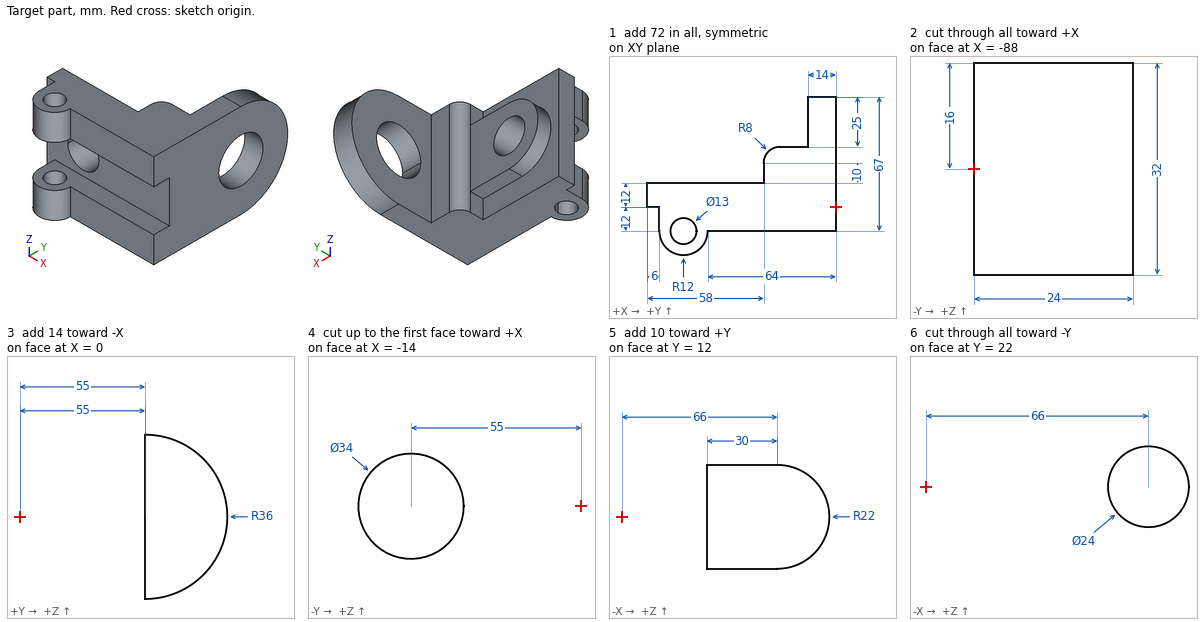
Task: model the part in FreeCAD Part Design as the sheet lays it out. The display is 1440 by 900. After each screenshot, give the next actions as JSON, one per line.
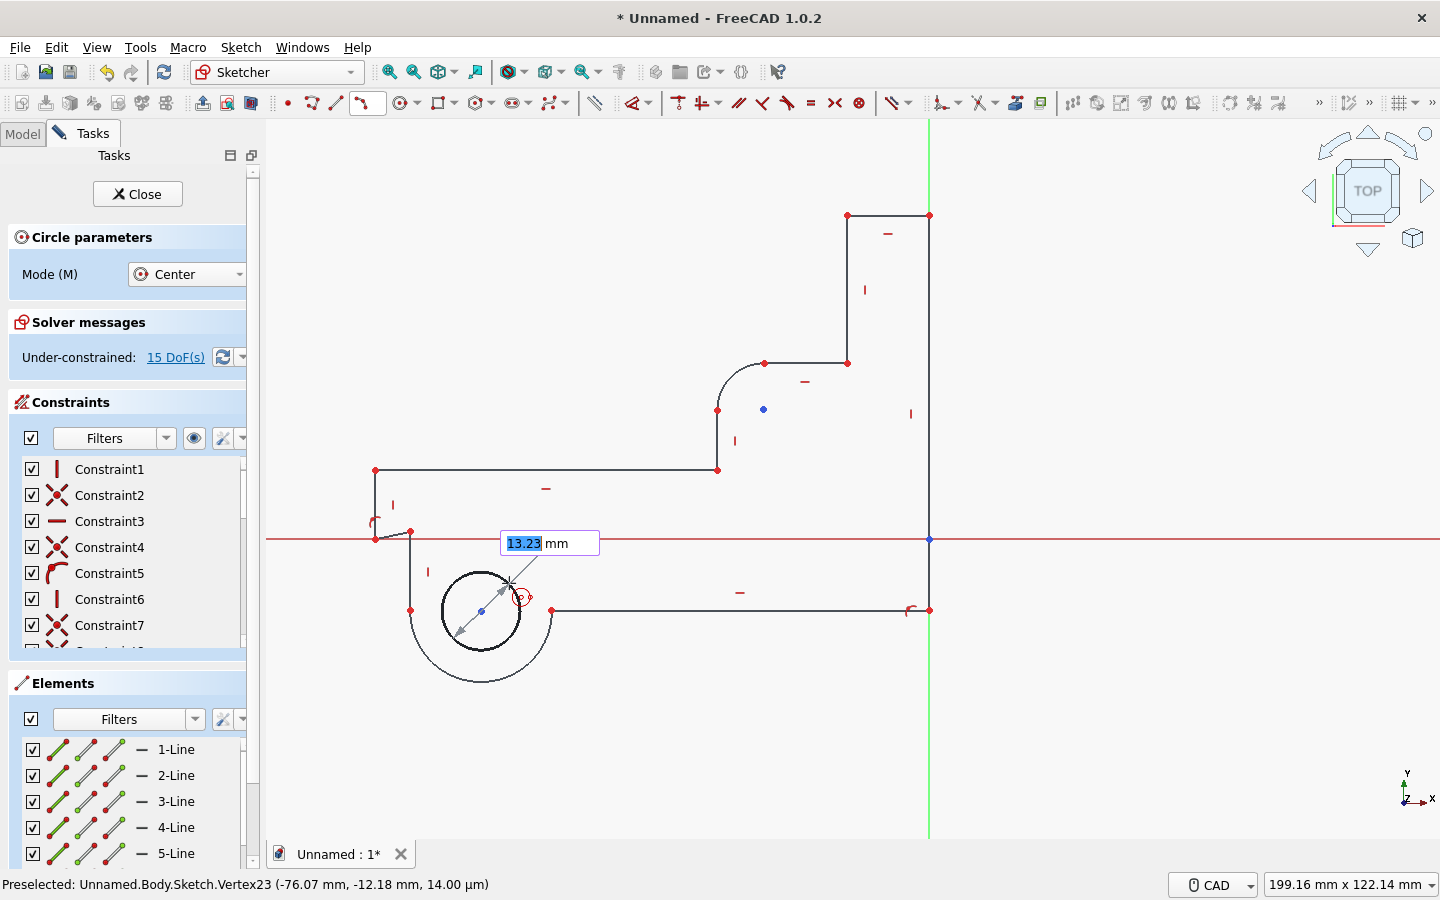
{"action": "type", "text": "13"}
{"action": "key", "text": "Return"}
{"action": "key", "text": "Escape"}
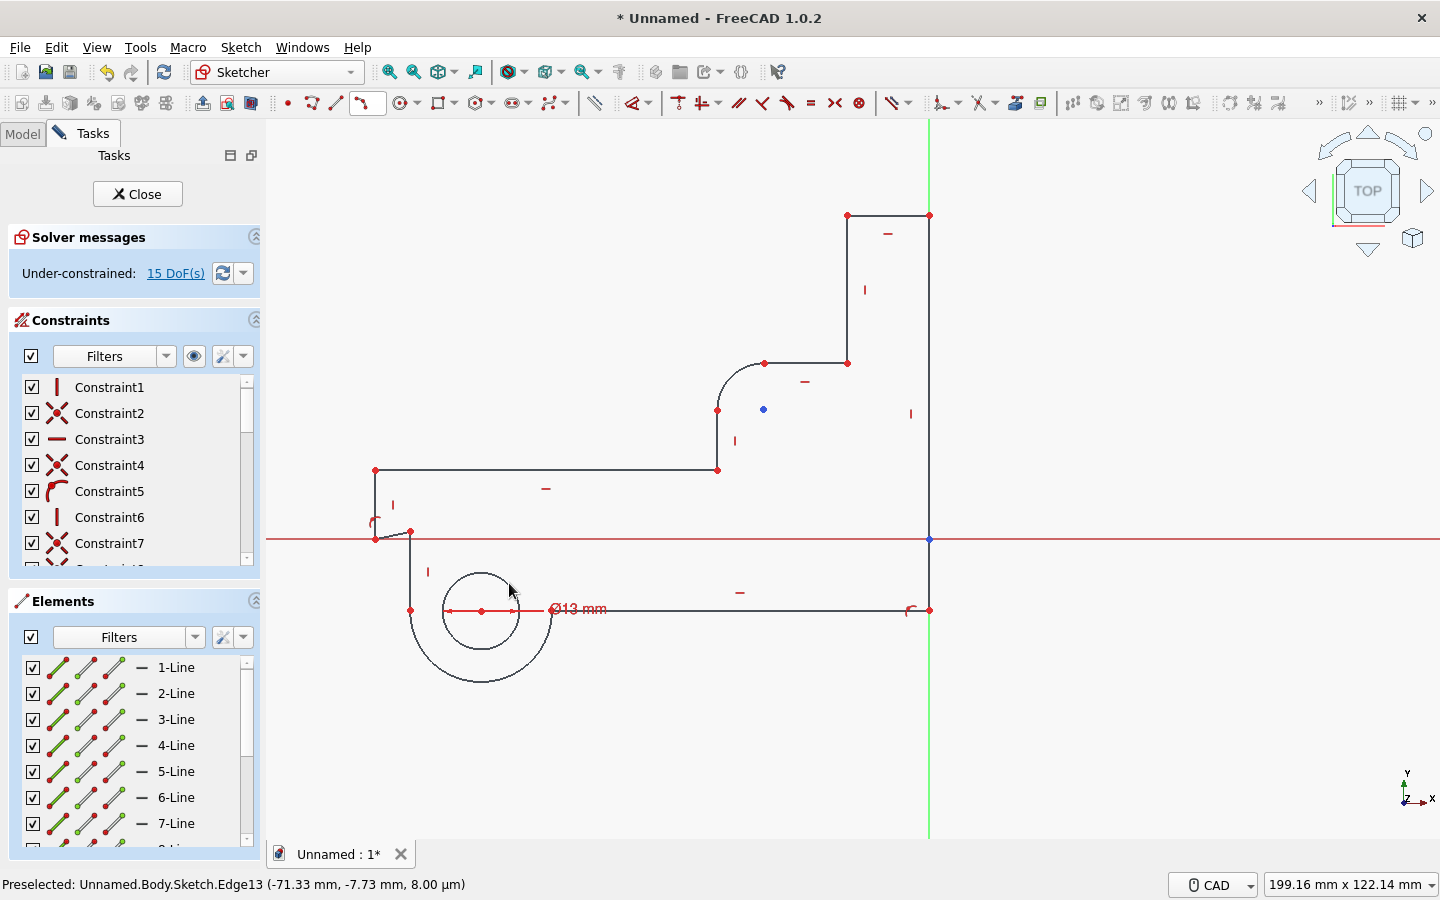
{"action": "left_click", "coordinate": [717, 428]}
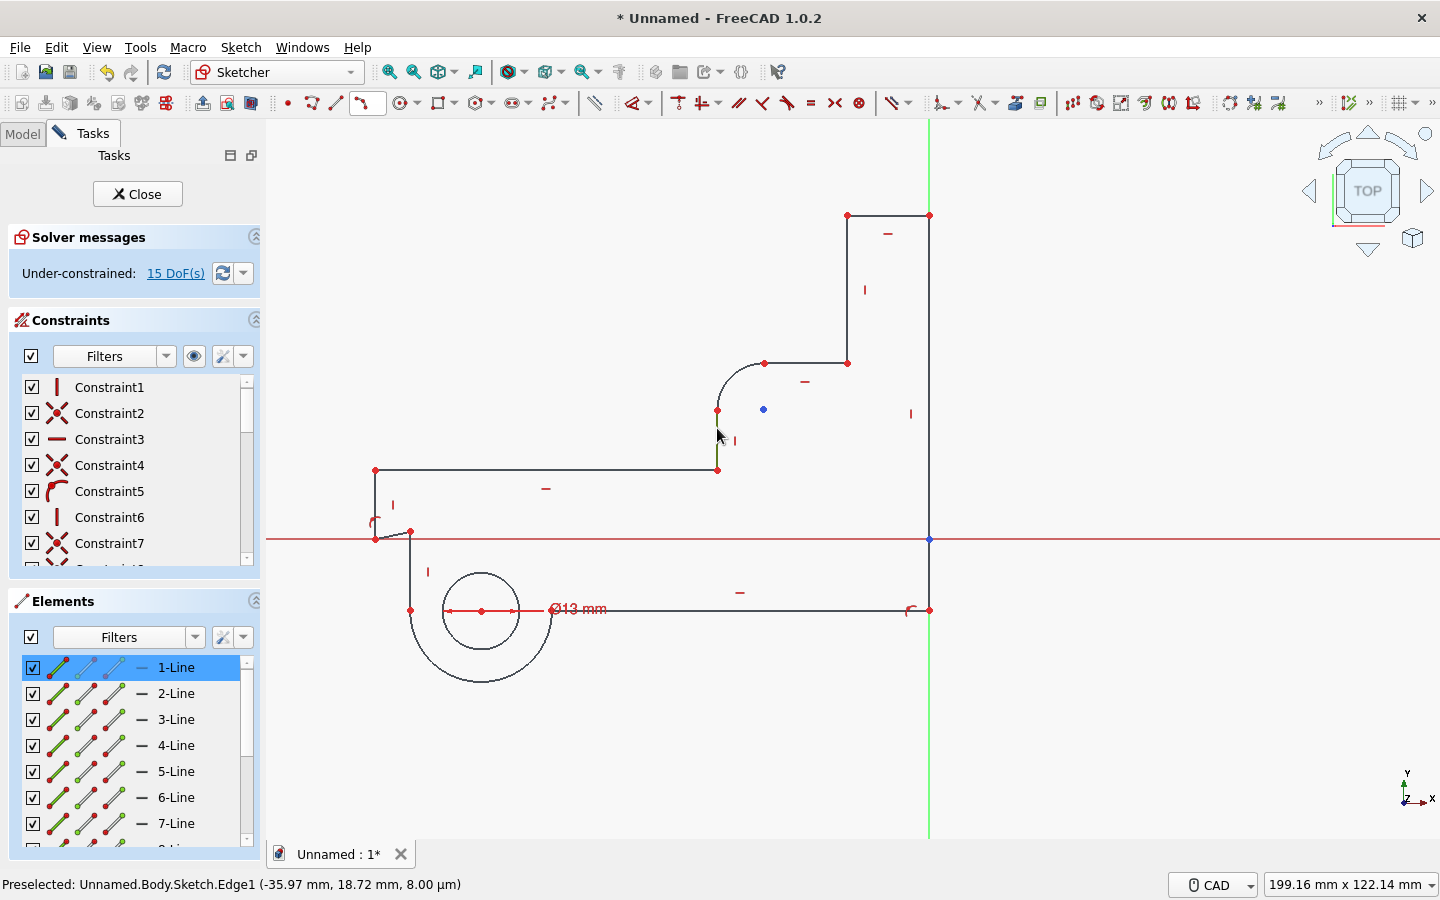
{"action": "left_click", "coordinate": [743, 368]}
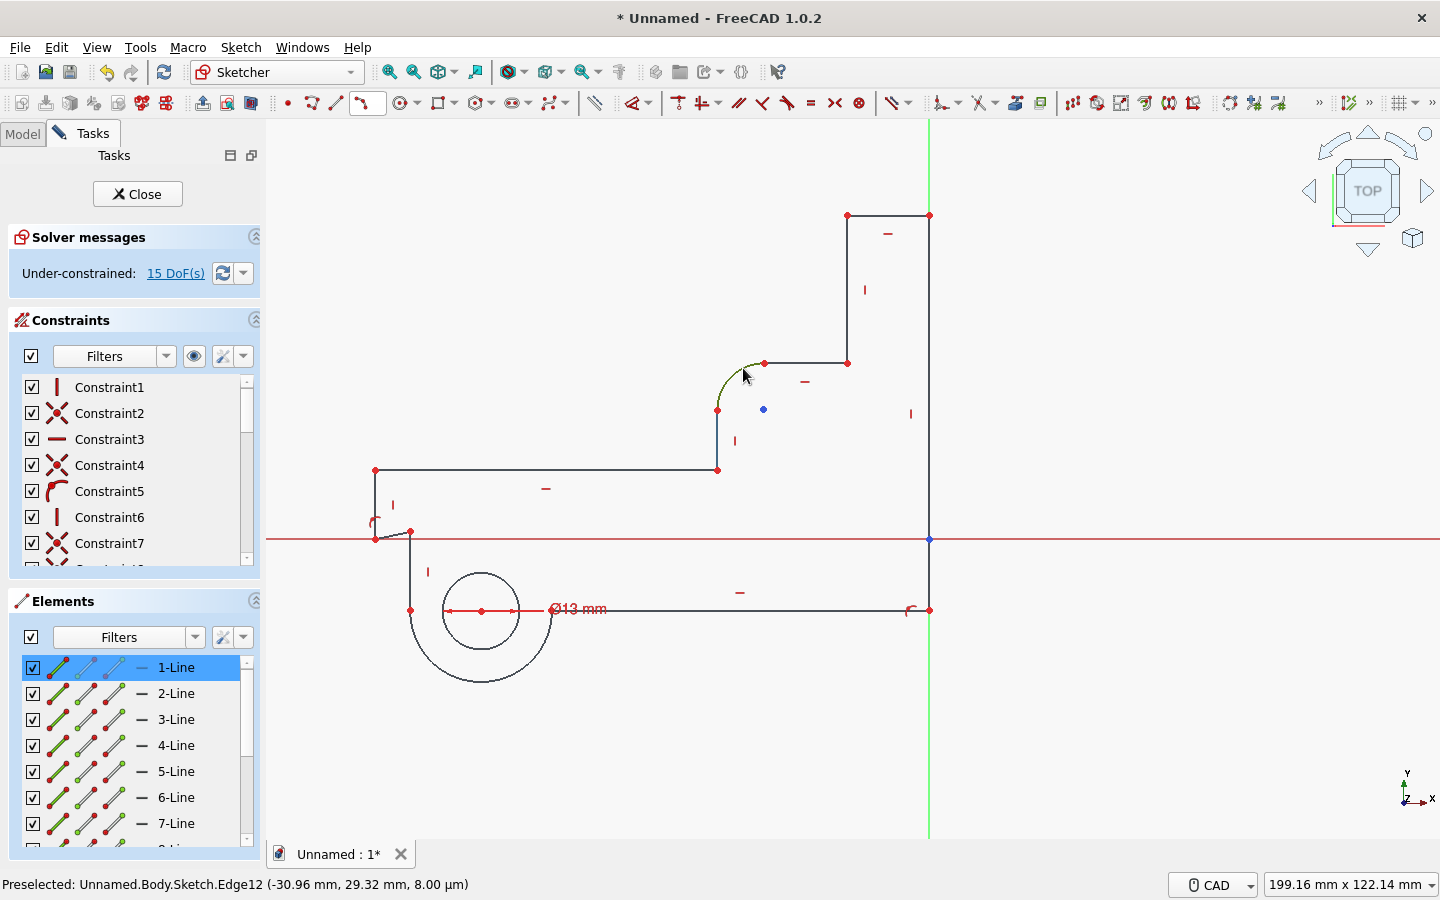
{"action": "left_click", "coordinate": [788, 104]}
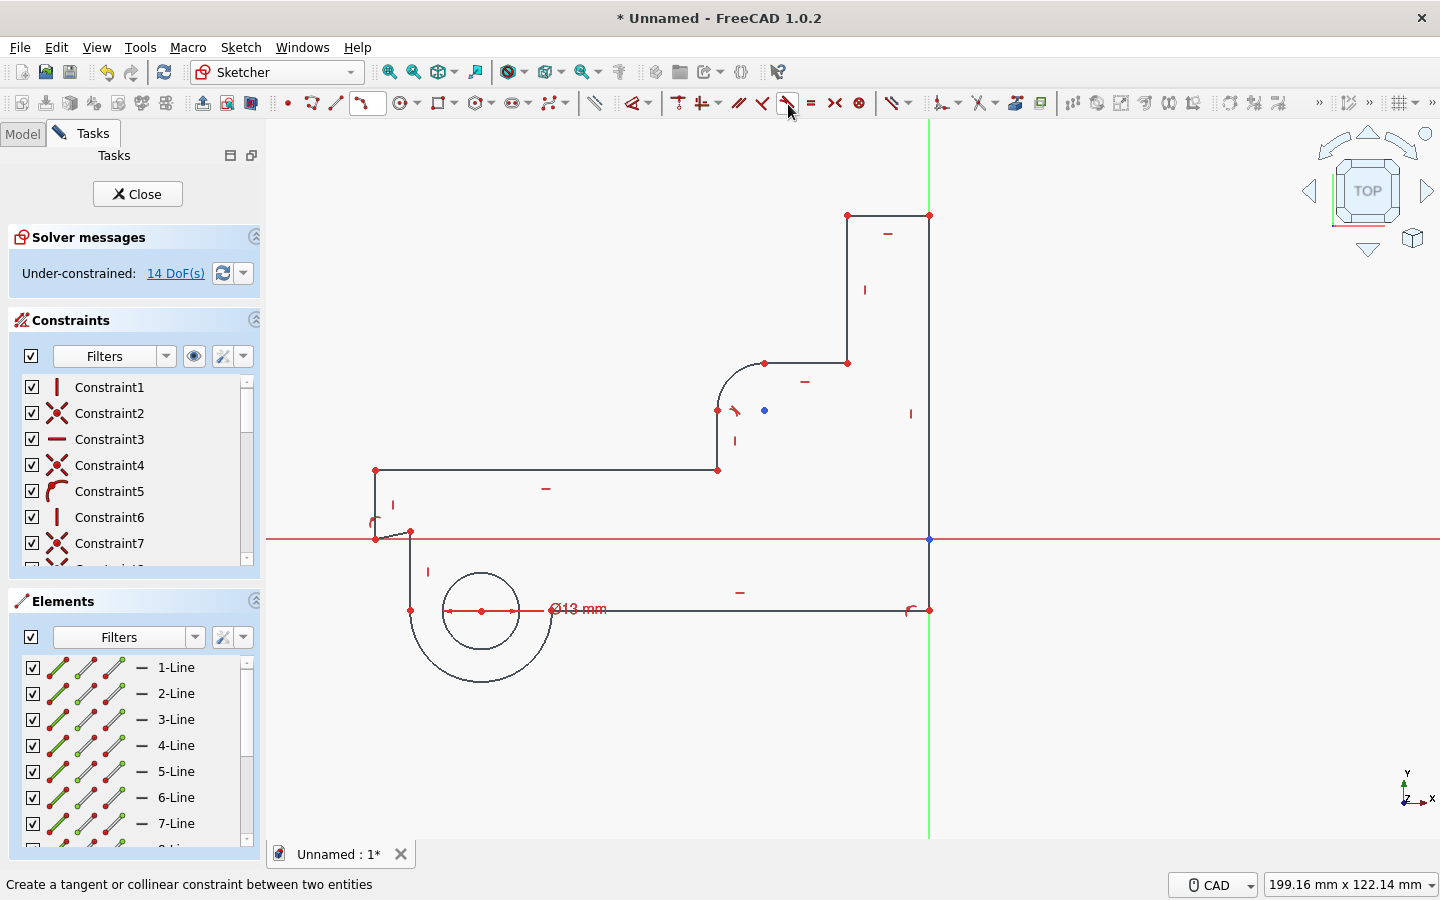
{"action": "left_click", "coordinate": [410, 555]}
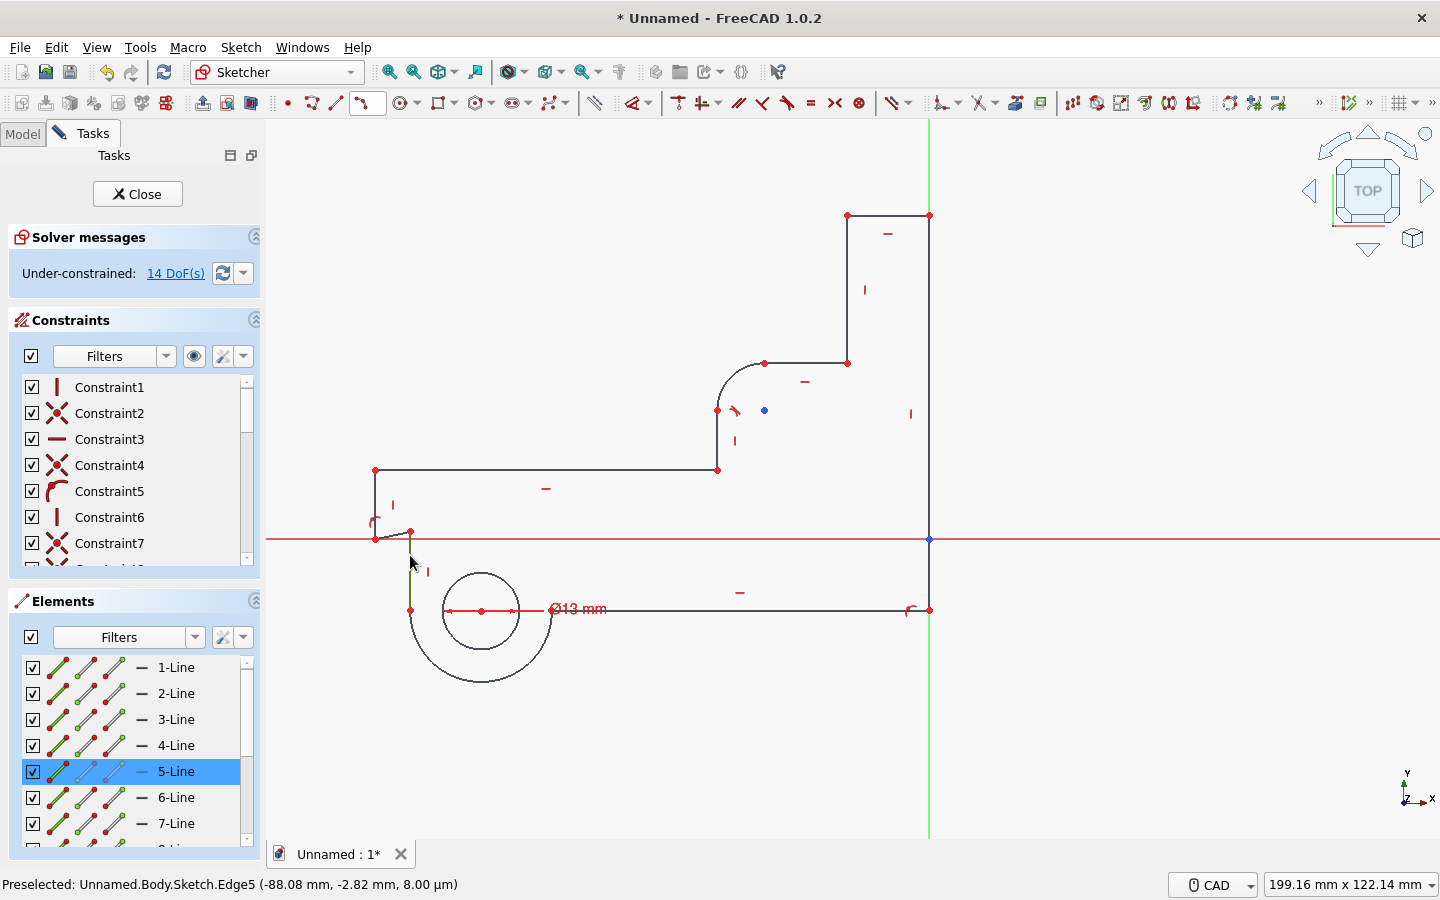
{"action": "left_click", "coordinate": [439, 668]}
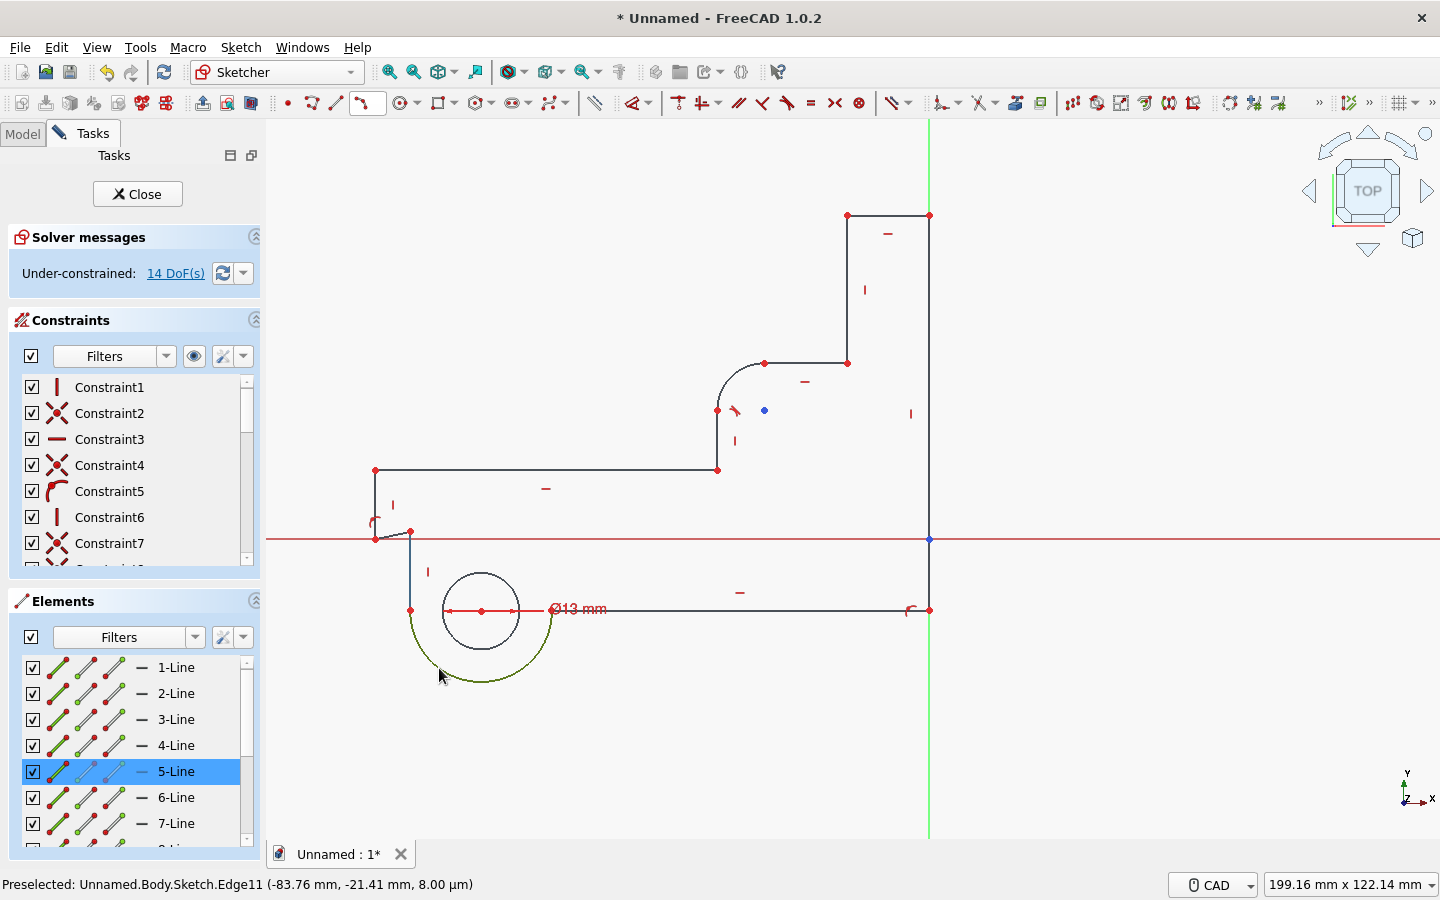
{"action": "left_click", "coordinate": [788, 104]}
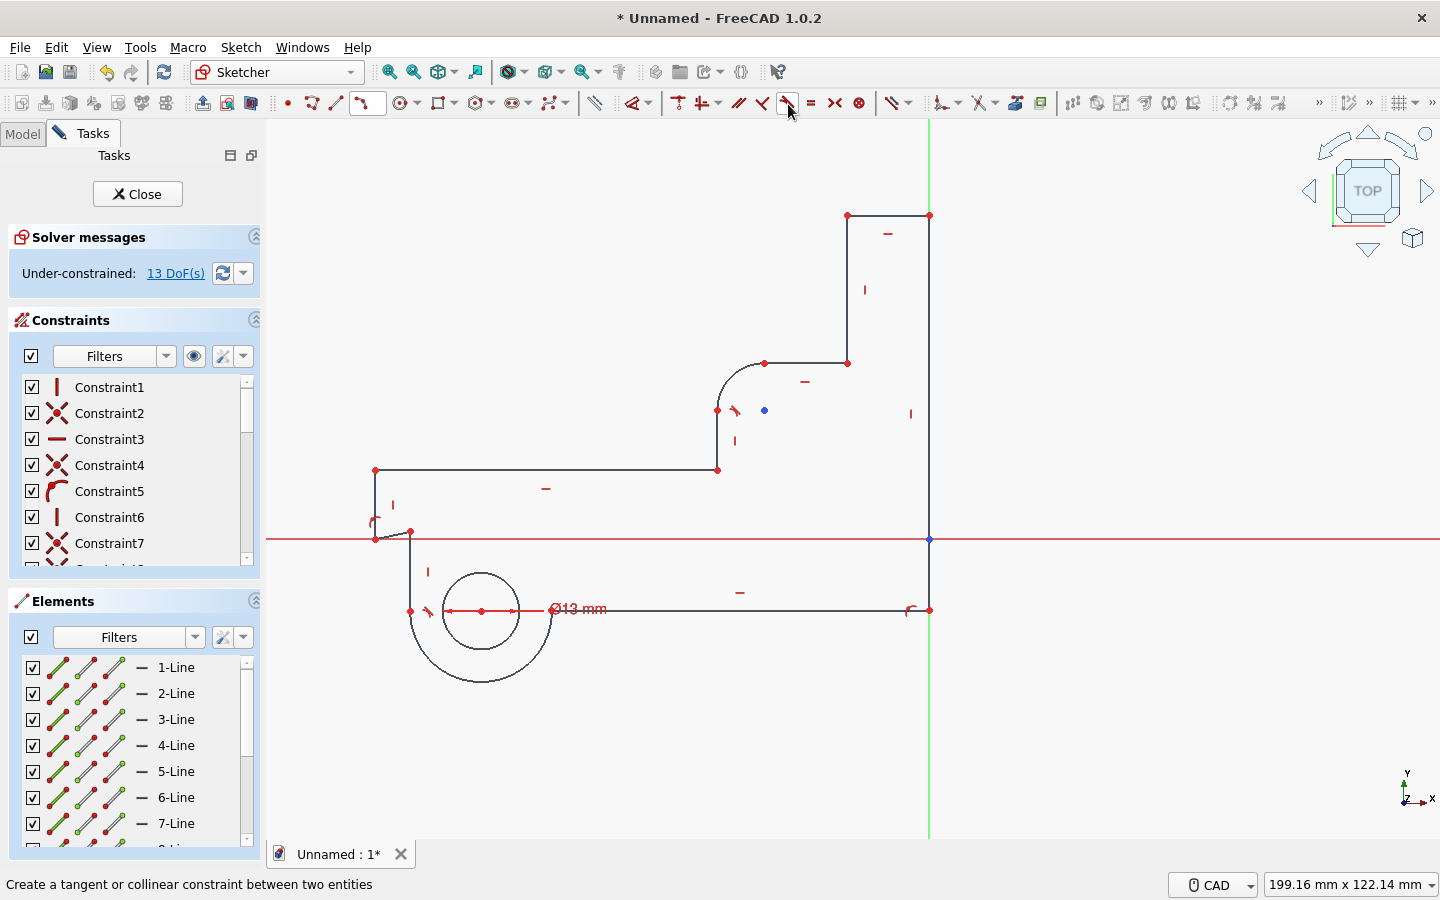
{"action": "left_click", "coordinate": [822, 363]}